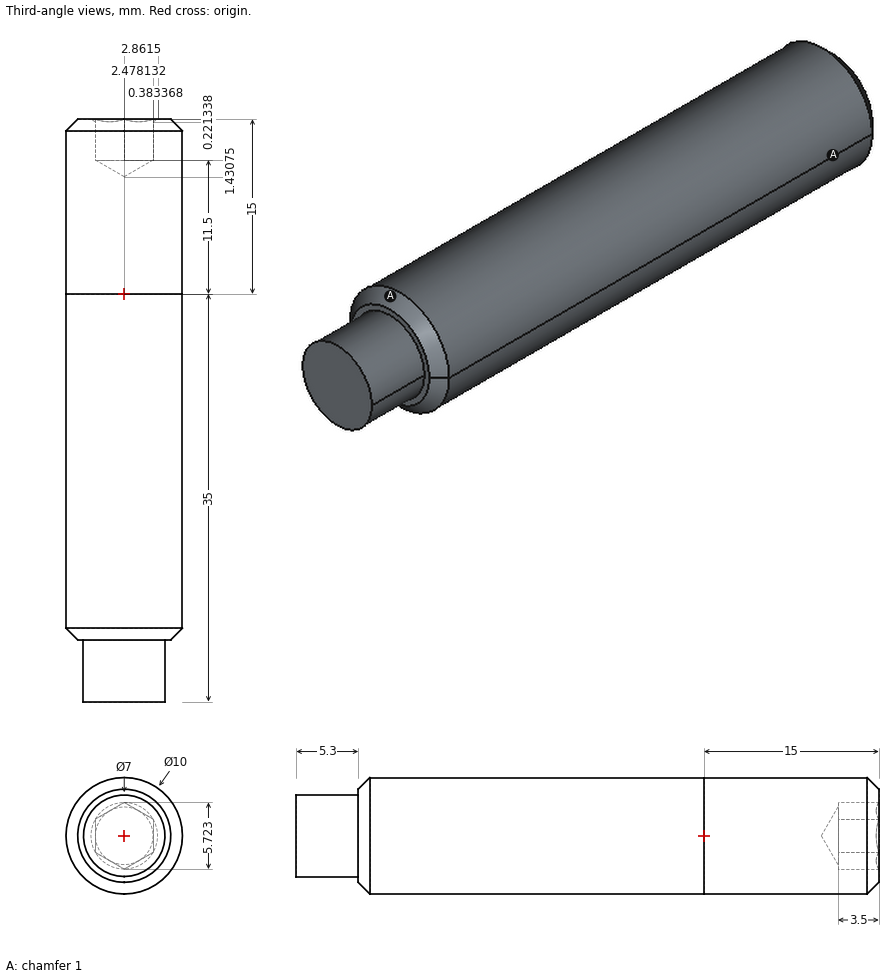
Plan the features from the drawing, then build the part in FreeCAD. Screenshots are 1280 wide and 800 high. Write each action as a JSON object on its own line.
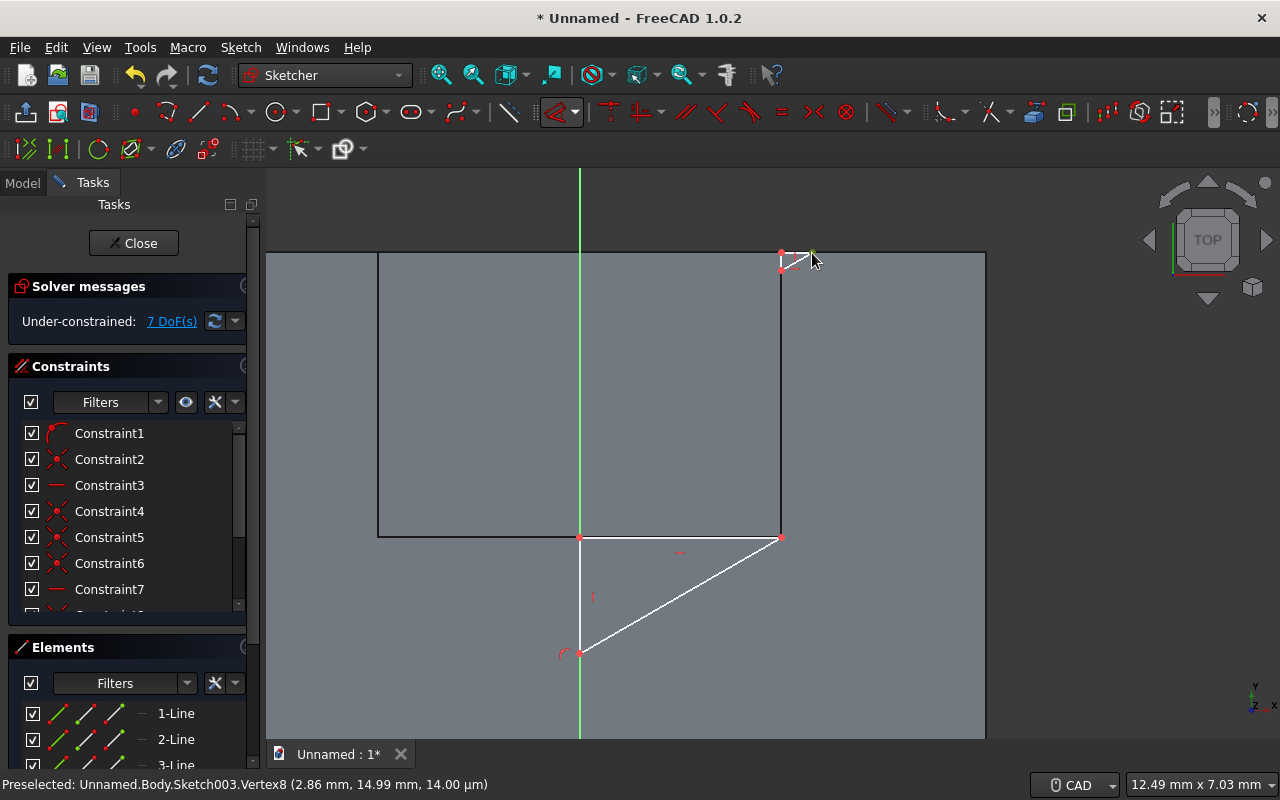
{"action": "left_click", "coordinate": [578, 112]}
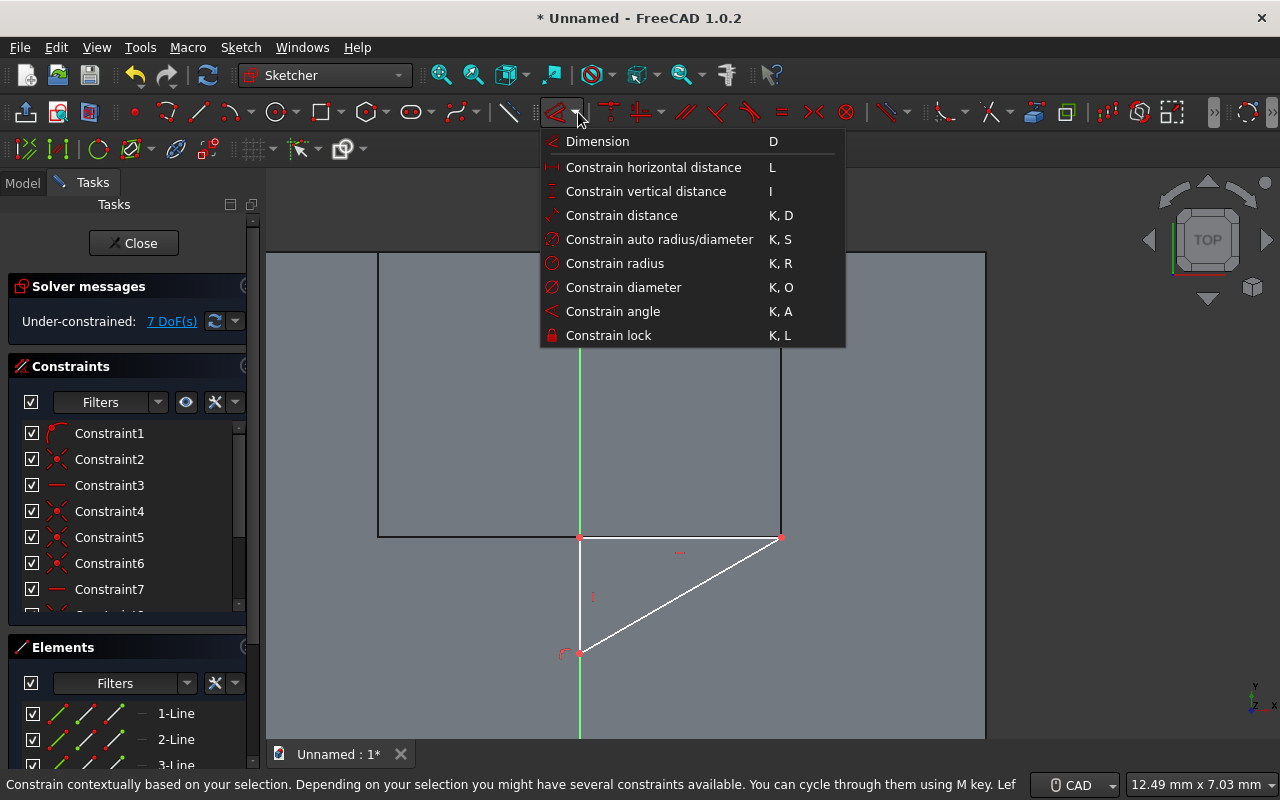
{"action": "left_click", "coordinate": [693, 191]}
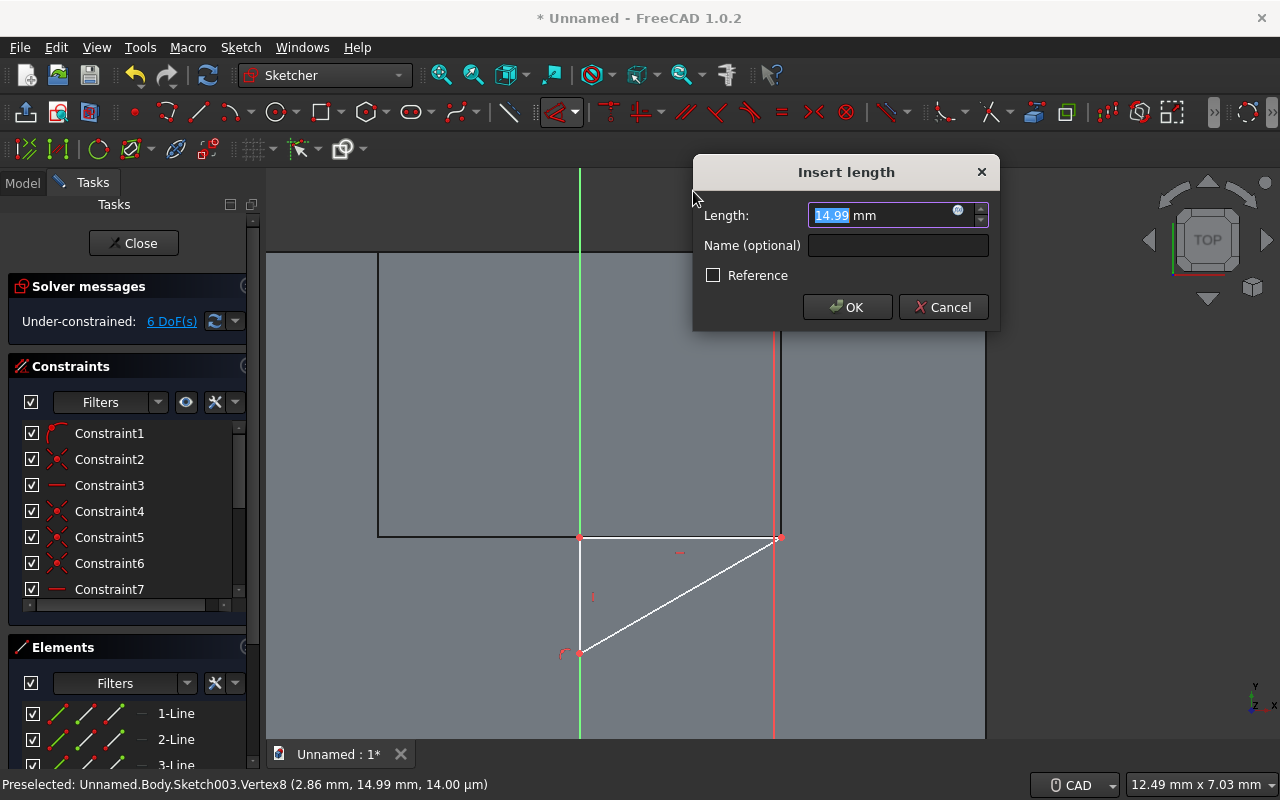
{"action": "type", "text": "15"}
{"action": "key", "text": "Return"}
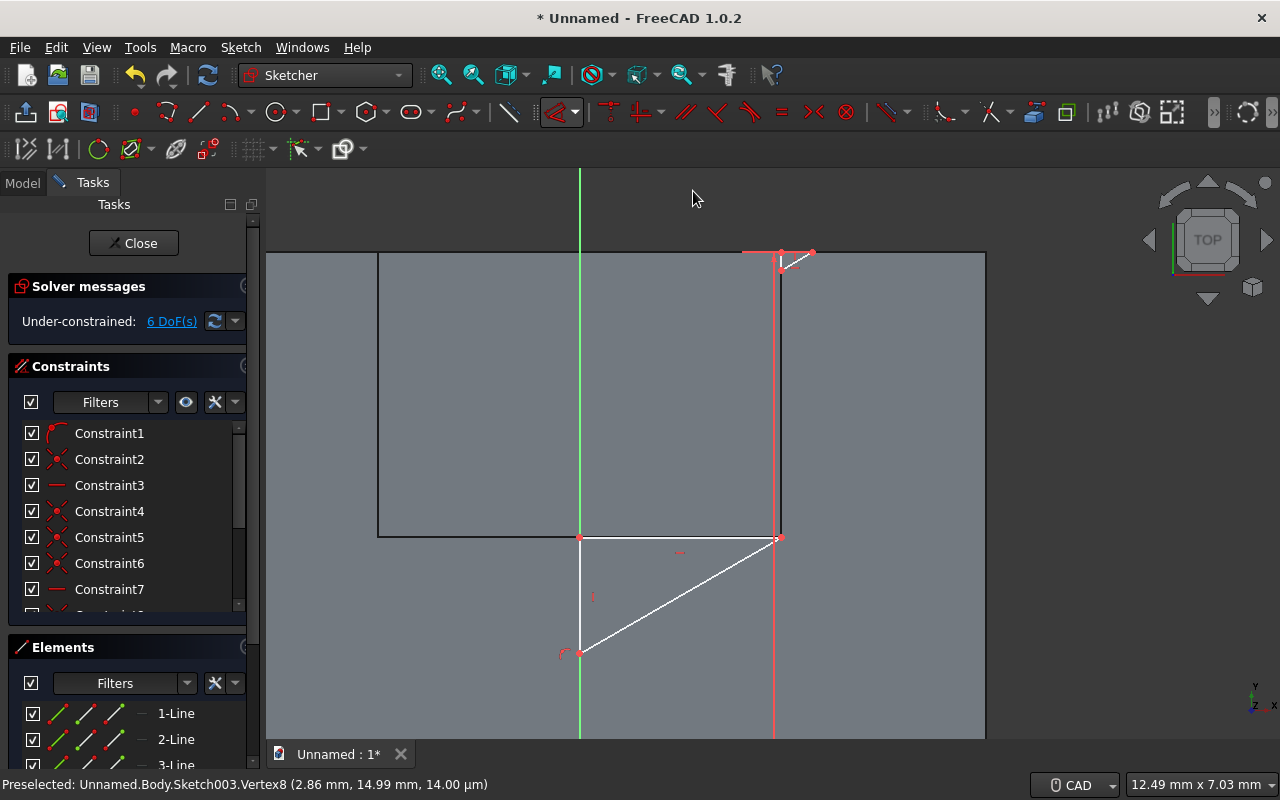
{"action": "left_click", "coordinate": [781, 538]}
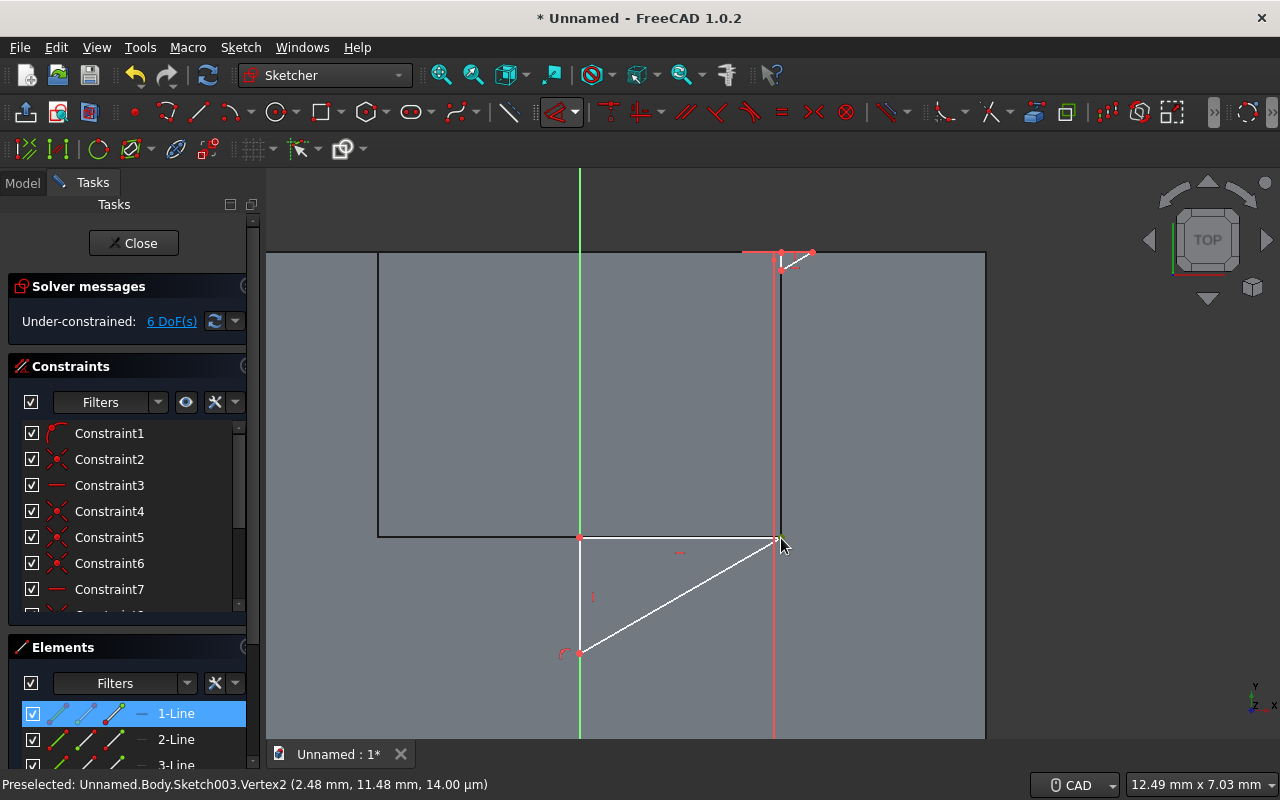
{"action": "key", "text": "i"}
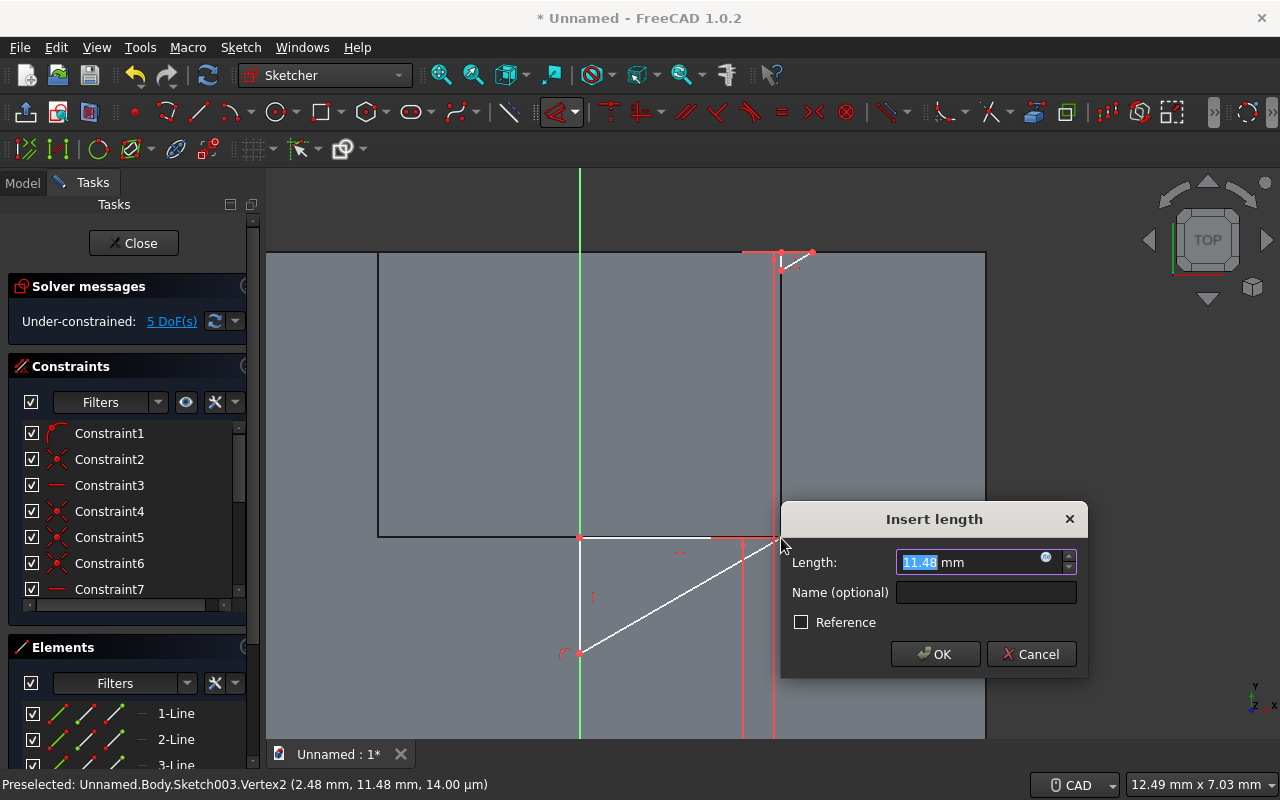
{"action": "type", "text": "11.5"}
{"action": "key", "text": "Return"}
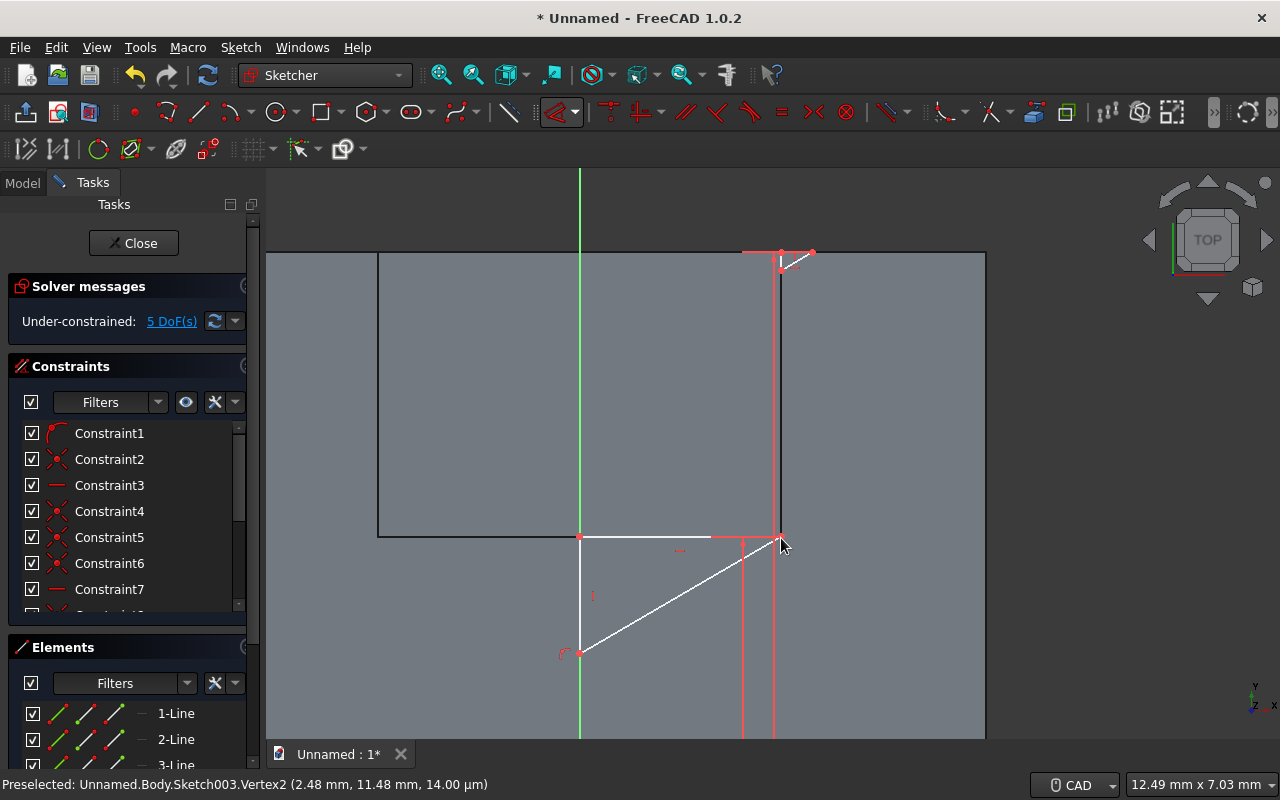
{"action": "left_click", "coordinate": [580, 572]}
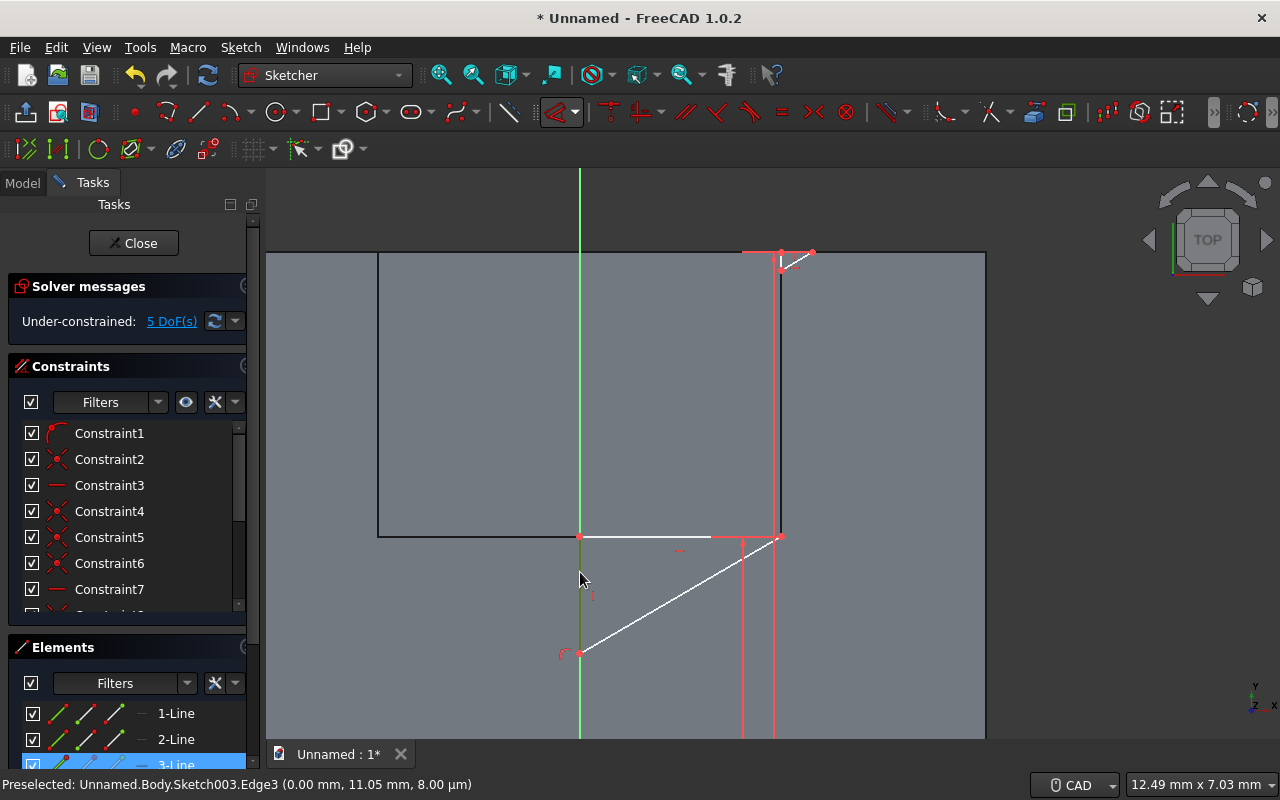
{"action": "left_click", "coordinate": [578, 112]}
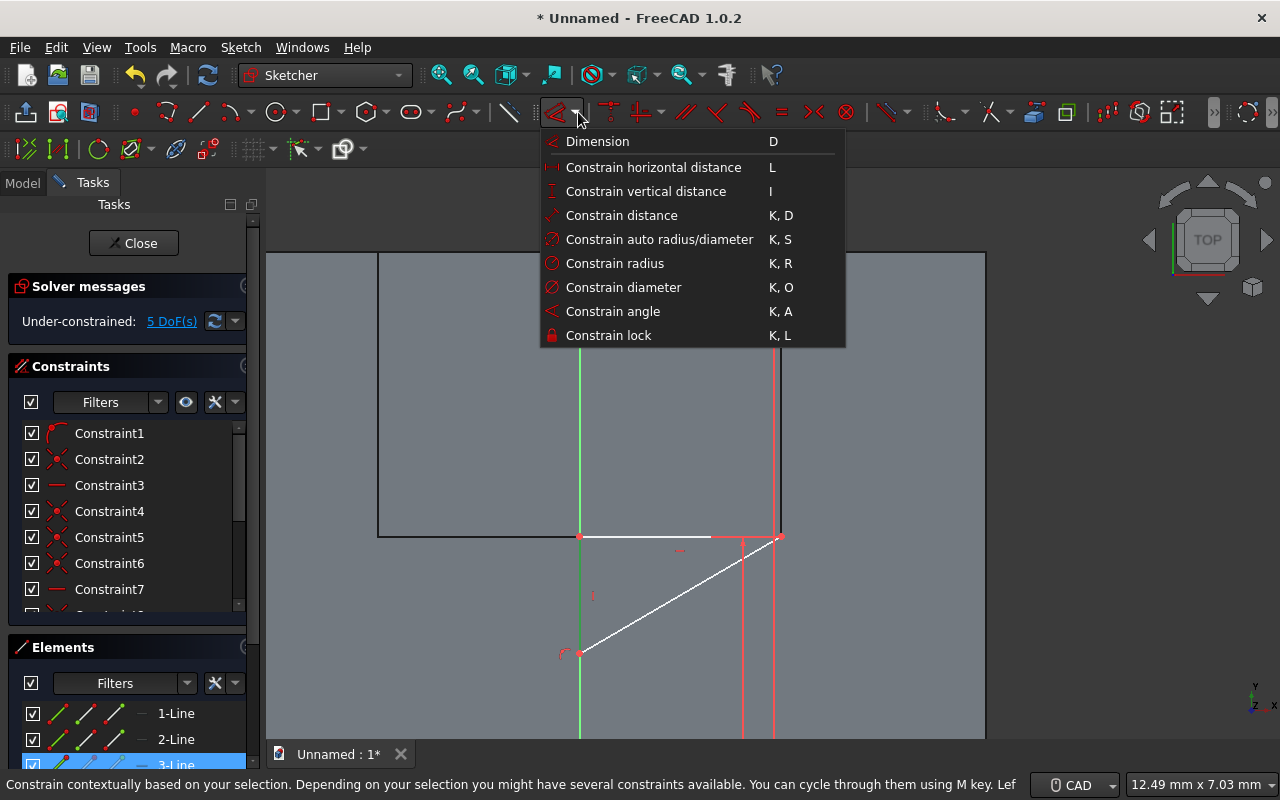
{"action": "left_click", "coordinate": [693, 191]}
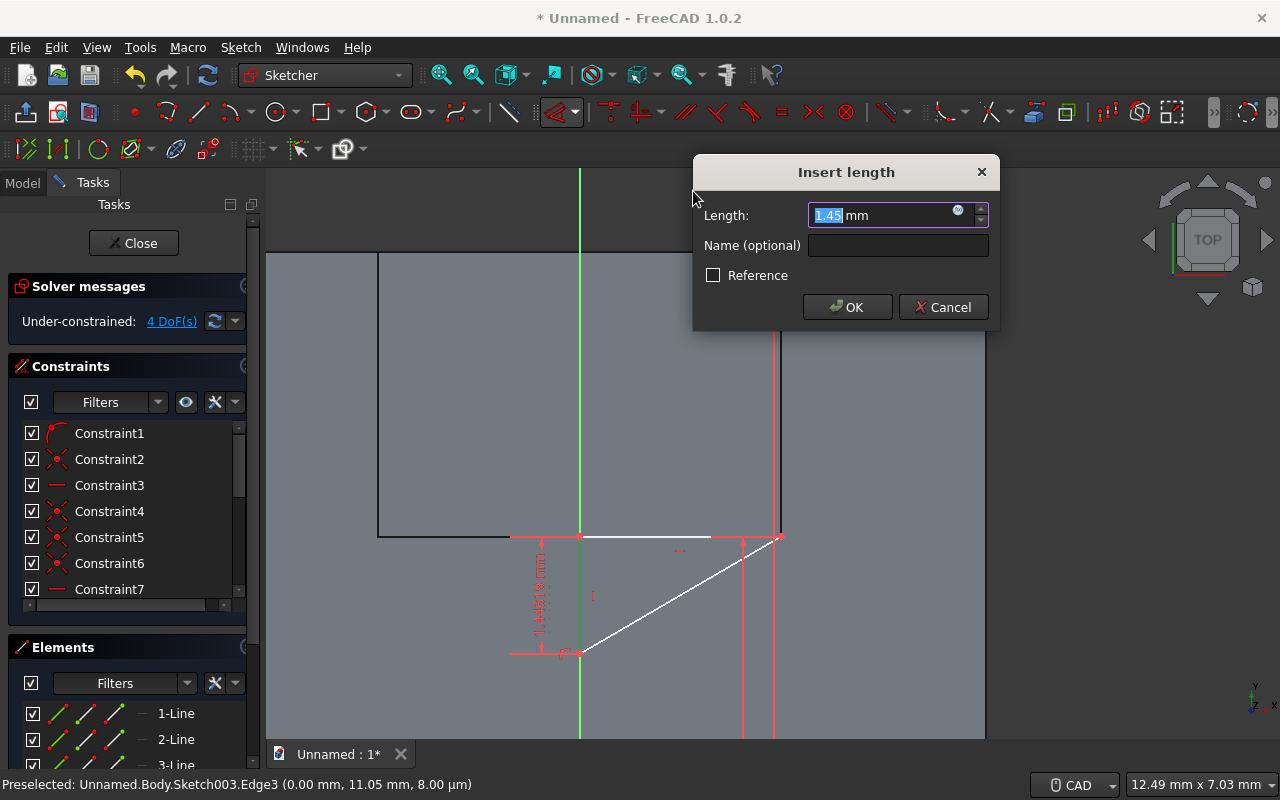
{"action": "type", "text": "1.43075"}
{"action": "key", "text": "Return"}